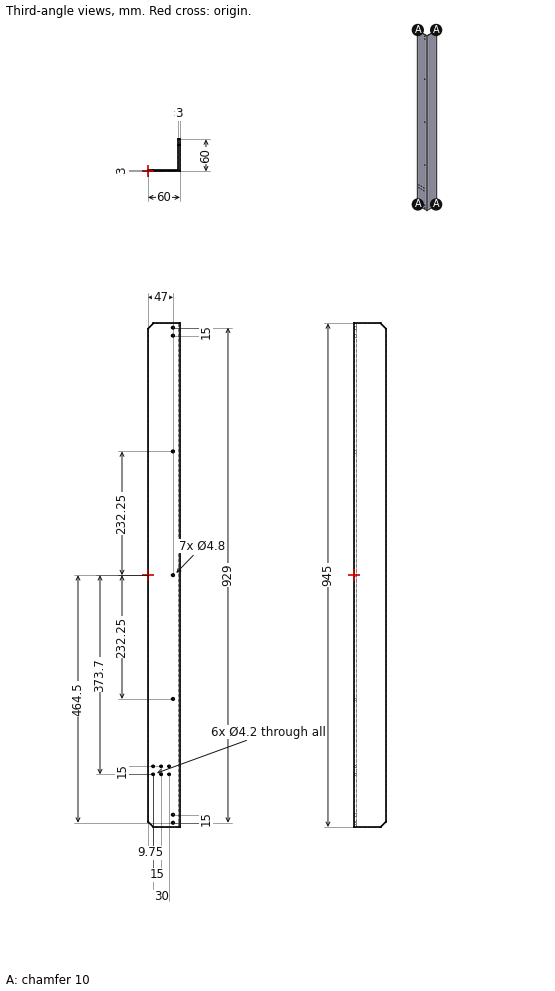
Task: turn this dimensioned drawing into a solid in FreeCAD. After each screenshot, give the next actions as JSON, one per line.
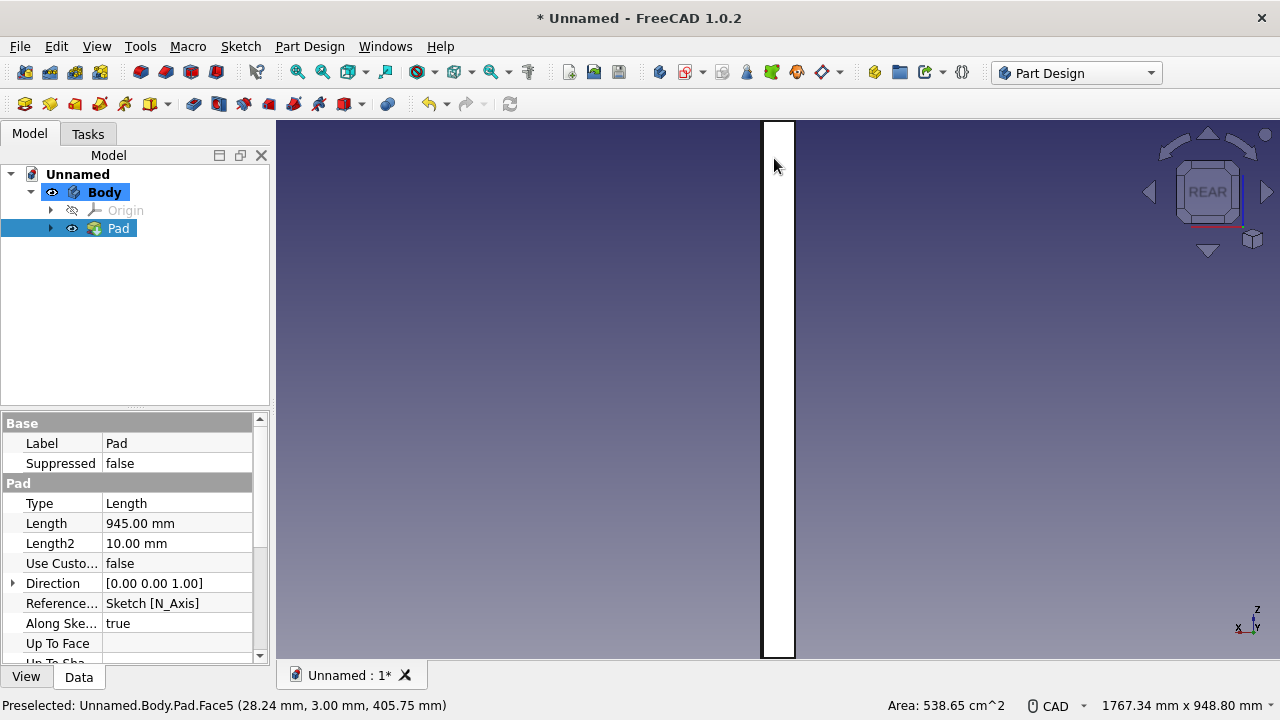
{"action": "left_click", "coordinate": [684, 72]}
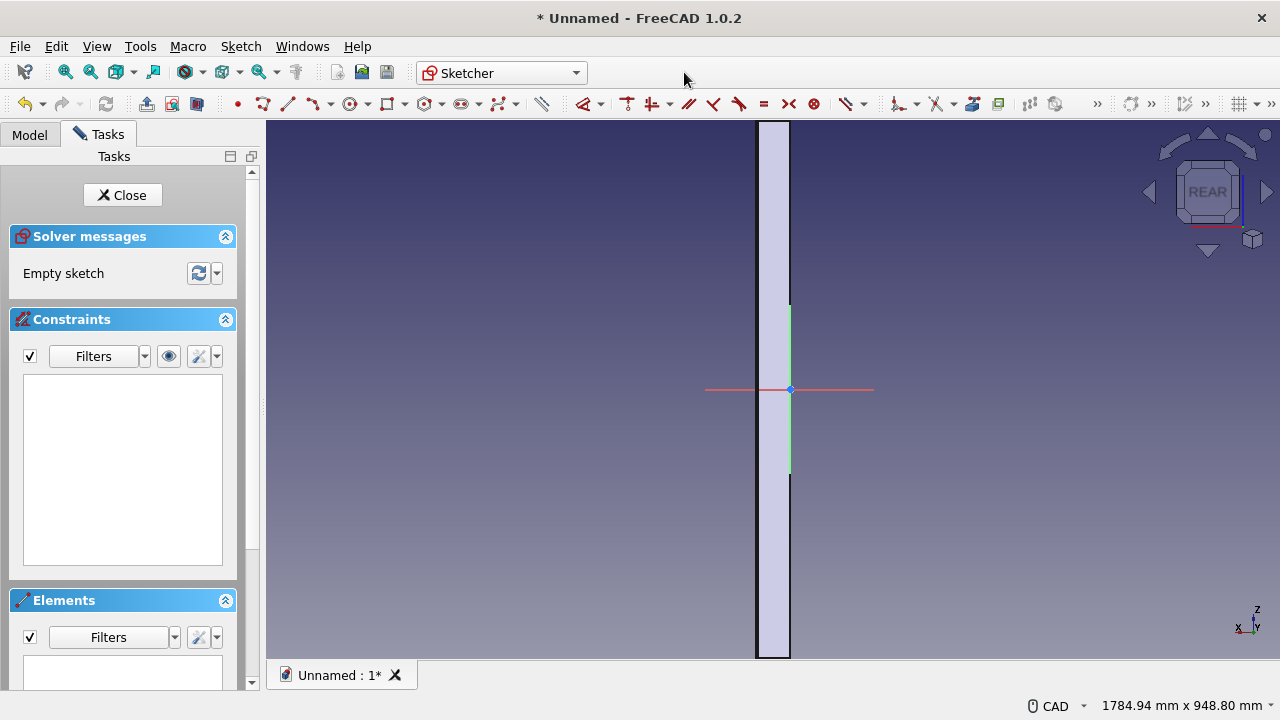
{"action": "left_click", "coordinate": [197, 104]}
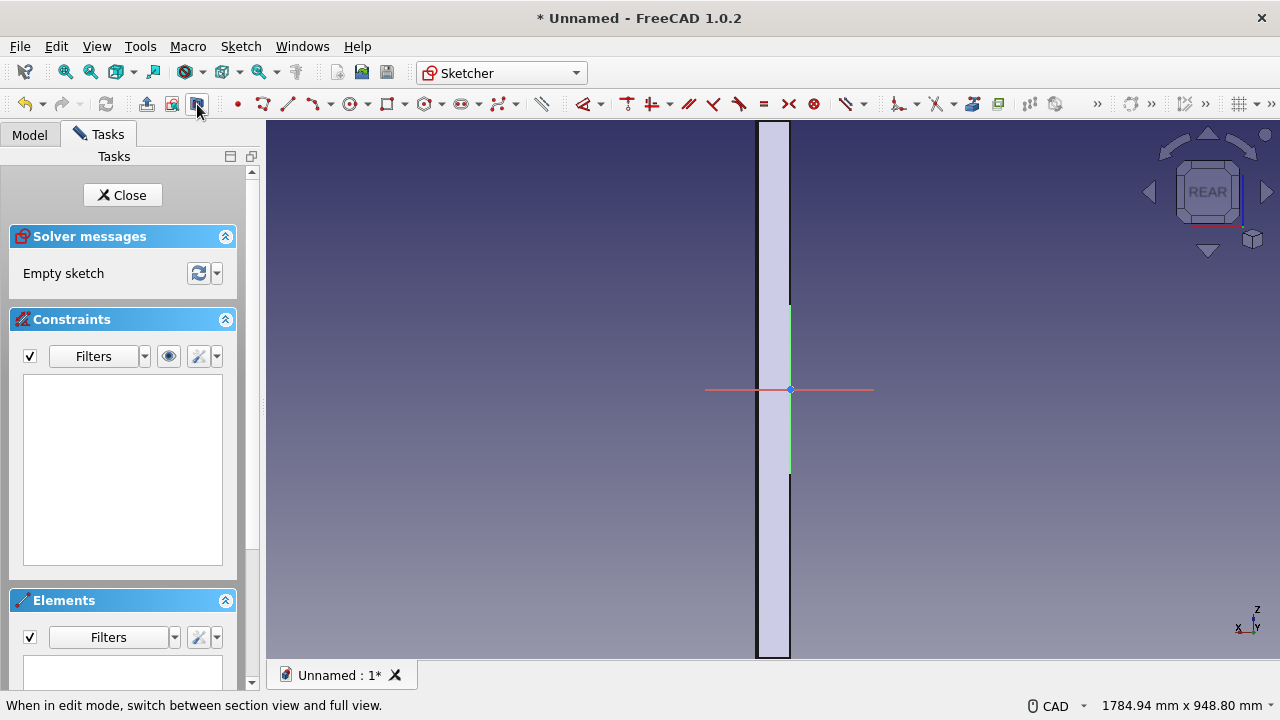
{"action": "scroll", "coordinate": [559, 390], "scroll_direction": "down", "scroll_amount": 2}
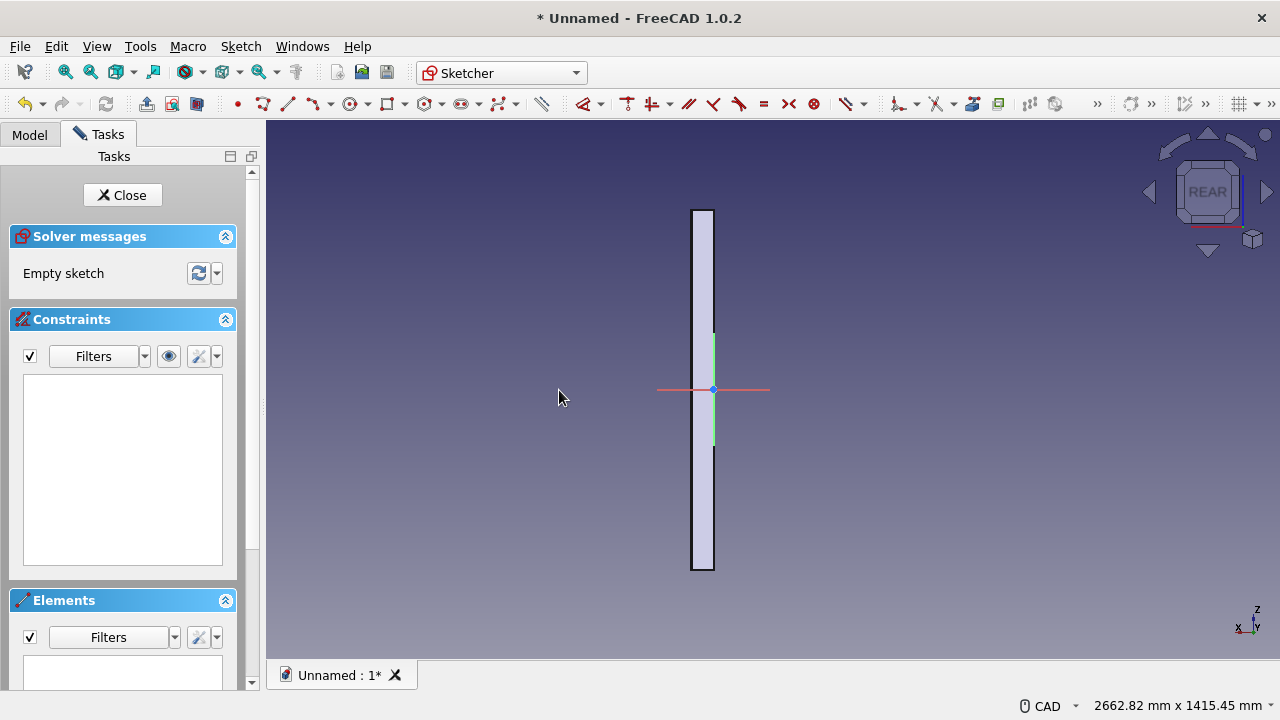
{"action": "left_click", "coordinate": [350, 104]}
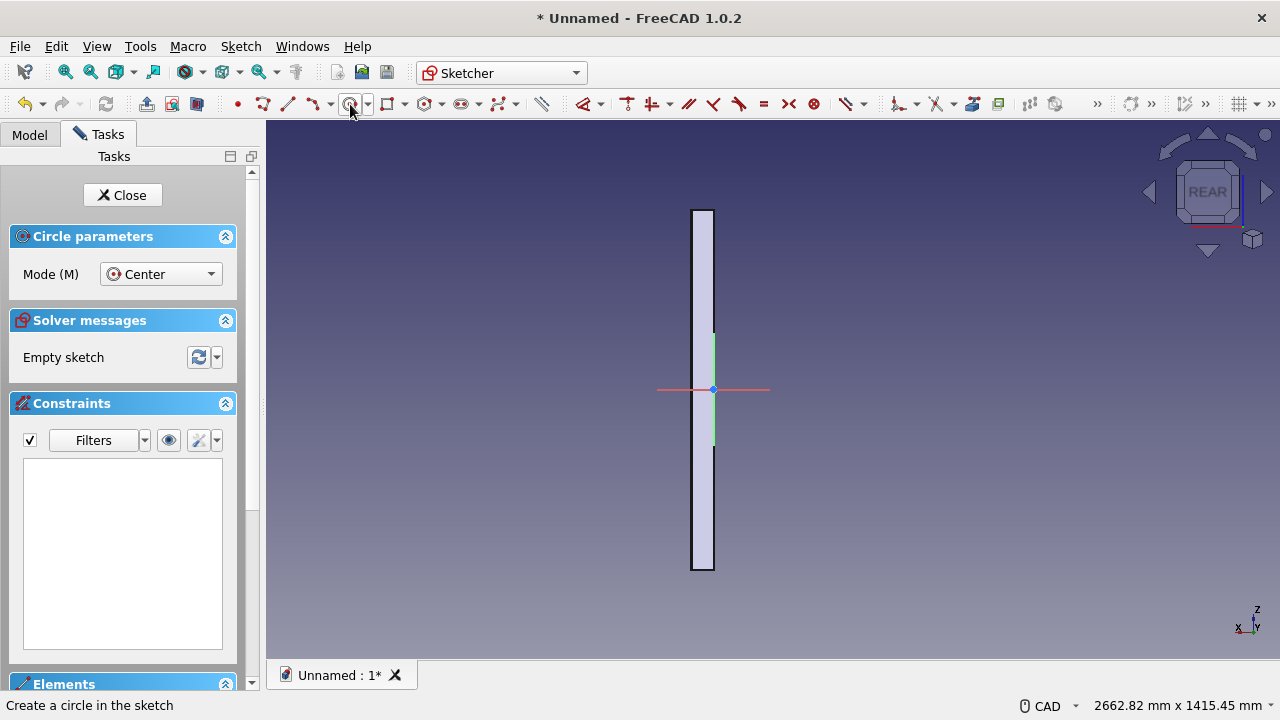
{"action": "scroll", "coordinate": [696, 390], "scroll_direction": "up", "scroll_amount": 17}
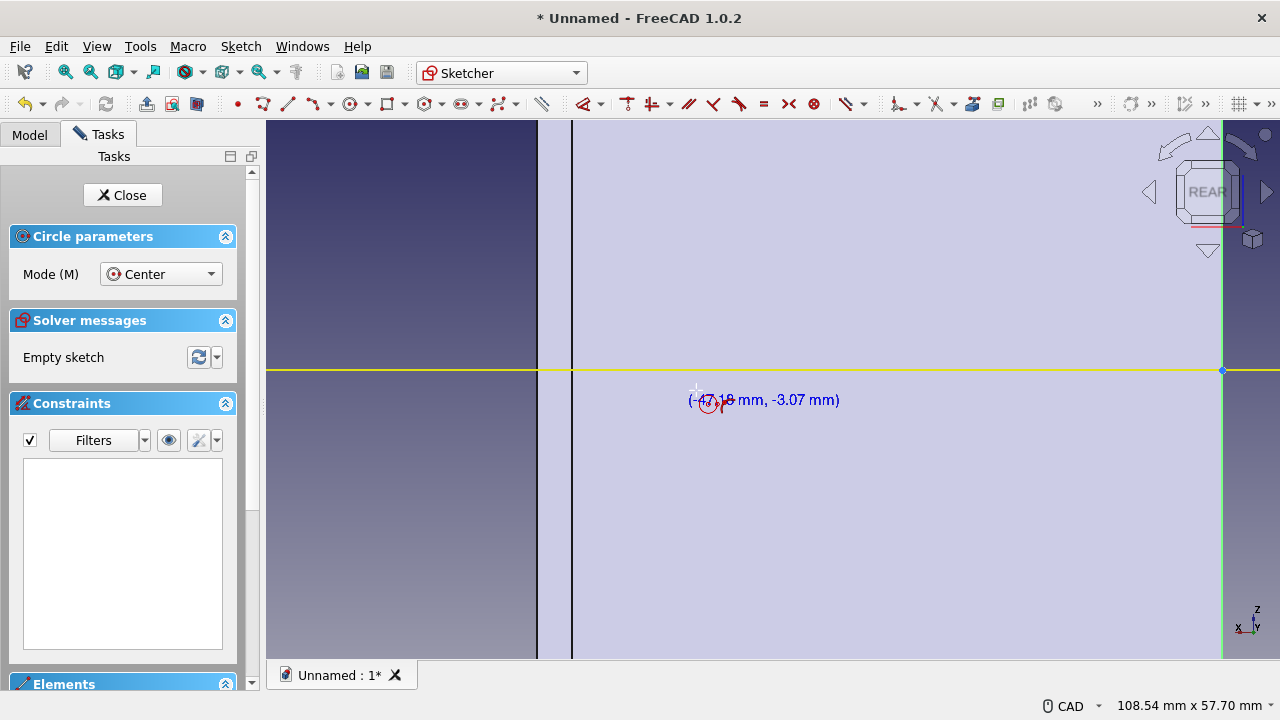
{"action": "scroll", "coordinate": [696, 390], "scroll_direction": "down", "scroll_amount": 17}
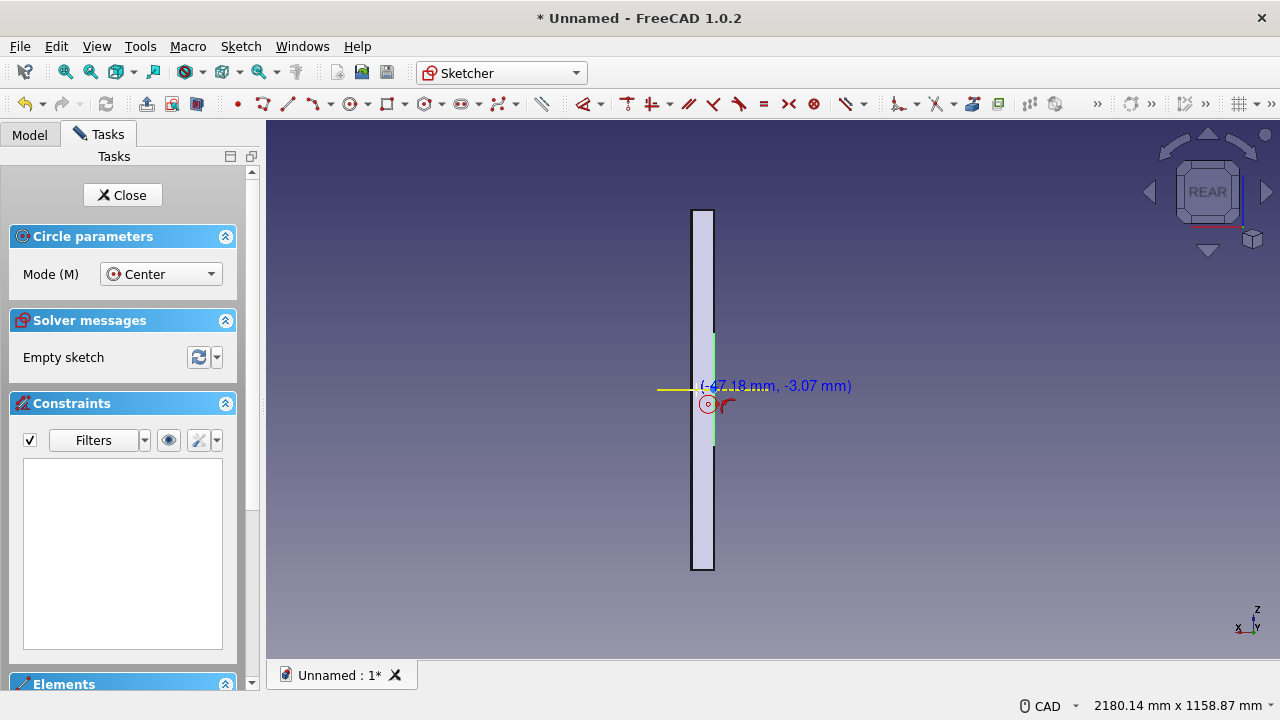
{"action": "left_click", "coordinate": [696, 390]}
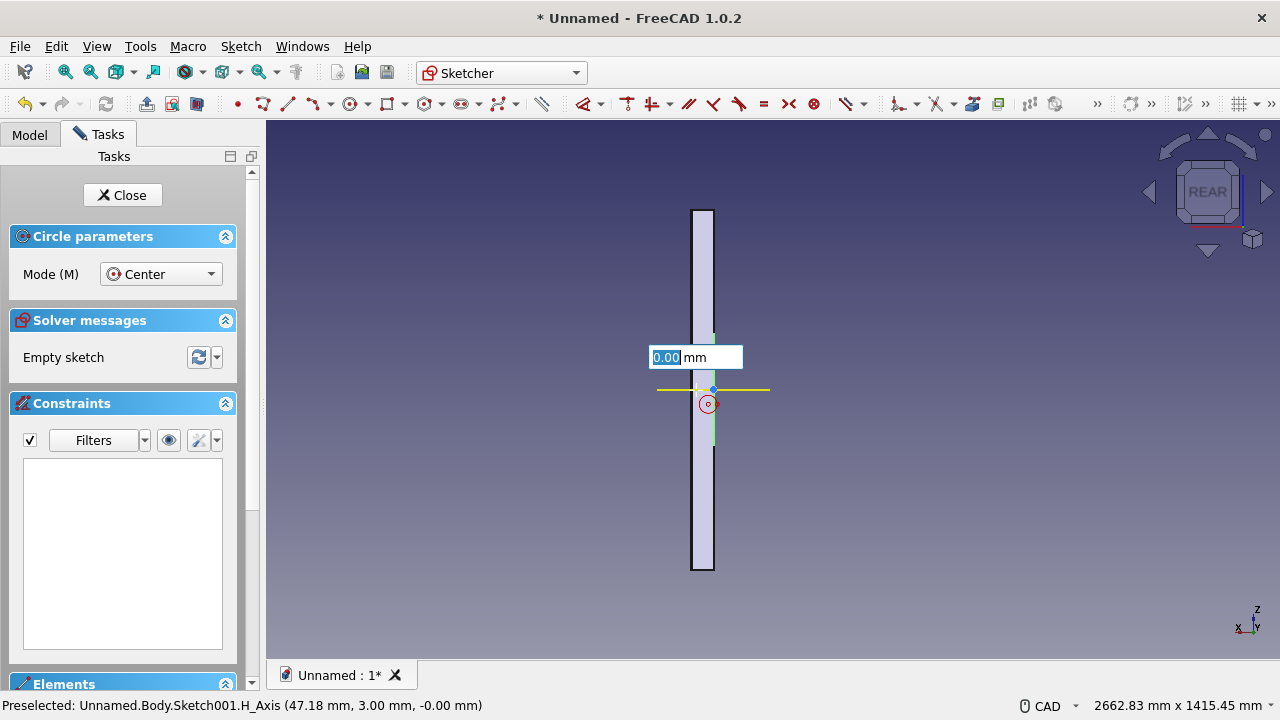
{"action": "scroll", "coordinate": [696, 389], "scroll_direction": "up", "scroll_amount": 15}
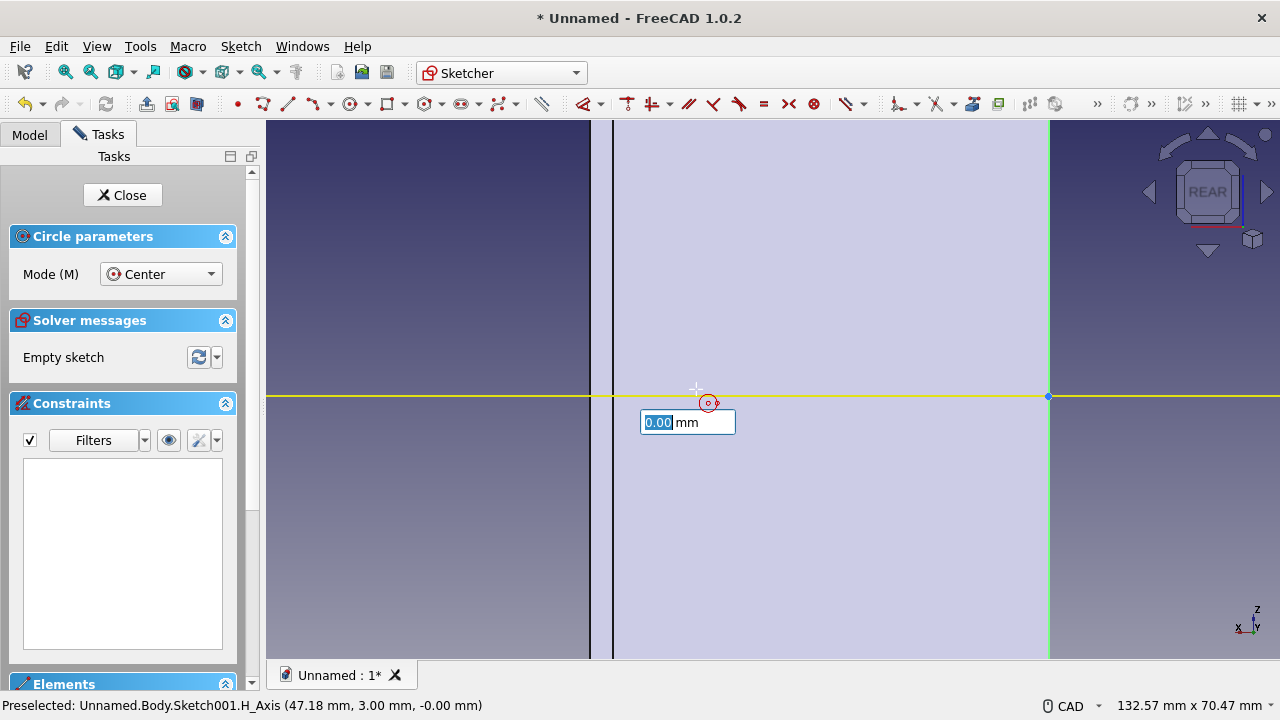
{"action": "left_click", "coordinate": [696, 379]}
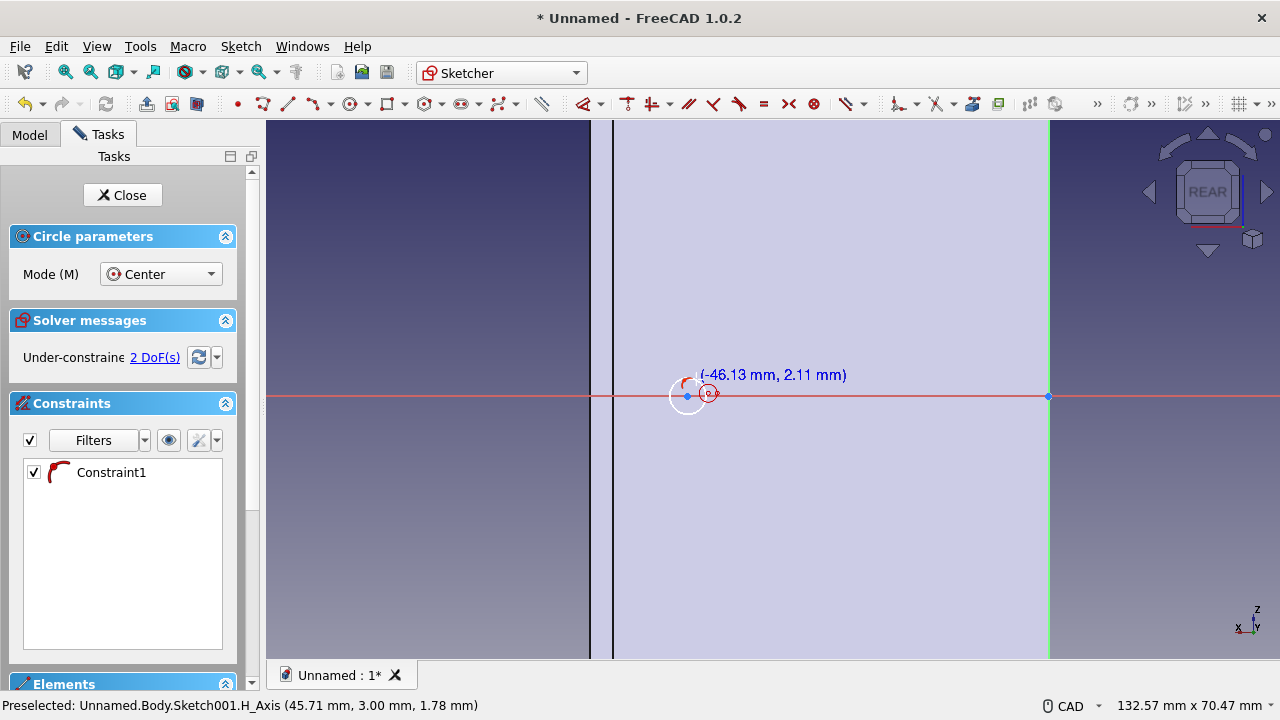
{"action": "scroll", "coordinate": [696, 389], "scroll_direction": "down", "scroll_amount": 15}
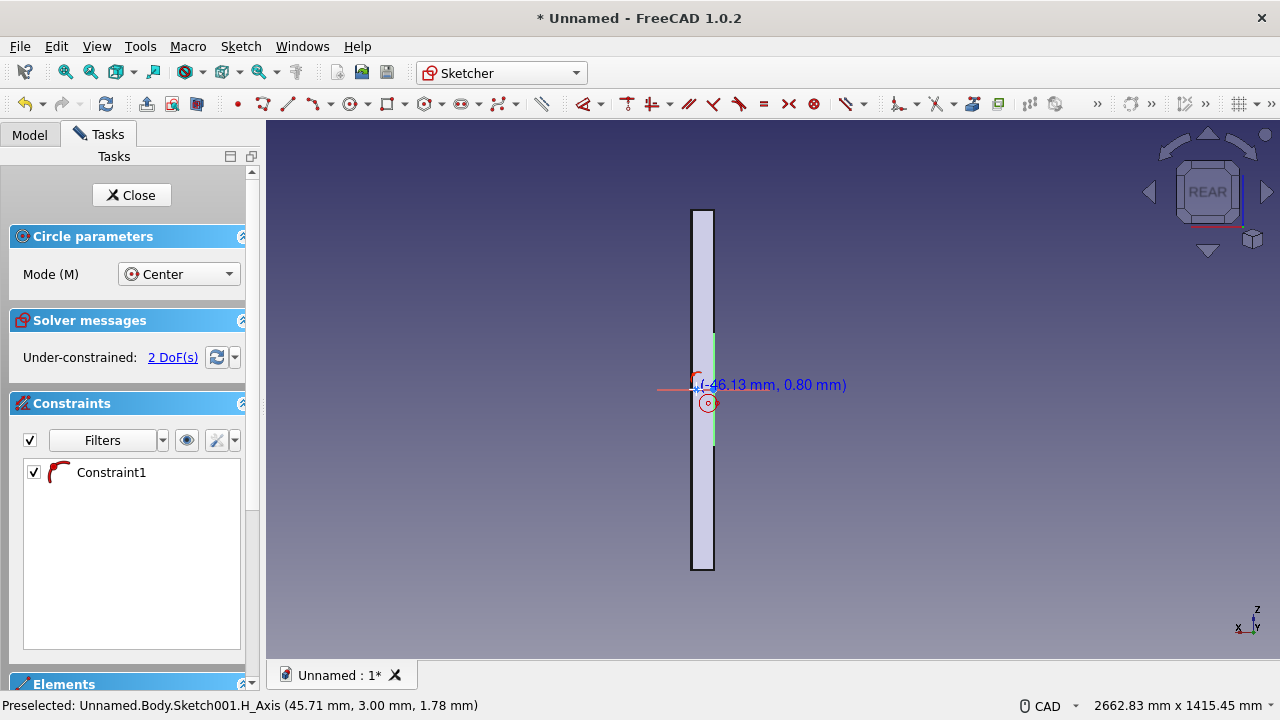
{"action": "scroll", "coordinate": [696, 478], "scroll_direction": "up", "scroll_amount": 17}